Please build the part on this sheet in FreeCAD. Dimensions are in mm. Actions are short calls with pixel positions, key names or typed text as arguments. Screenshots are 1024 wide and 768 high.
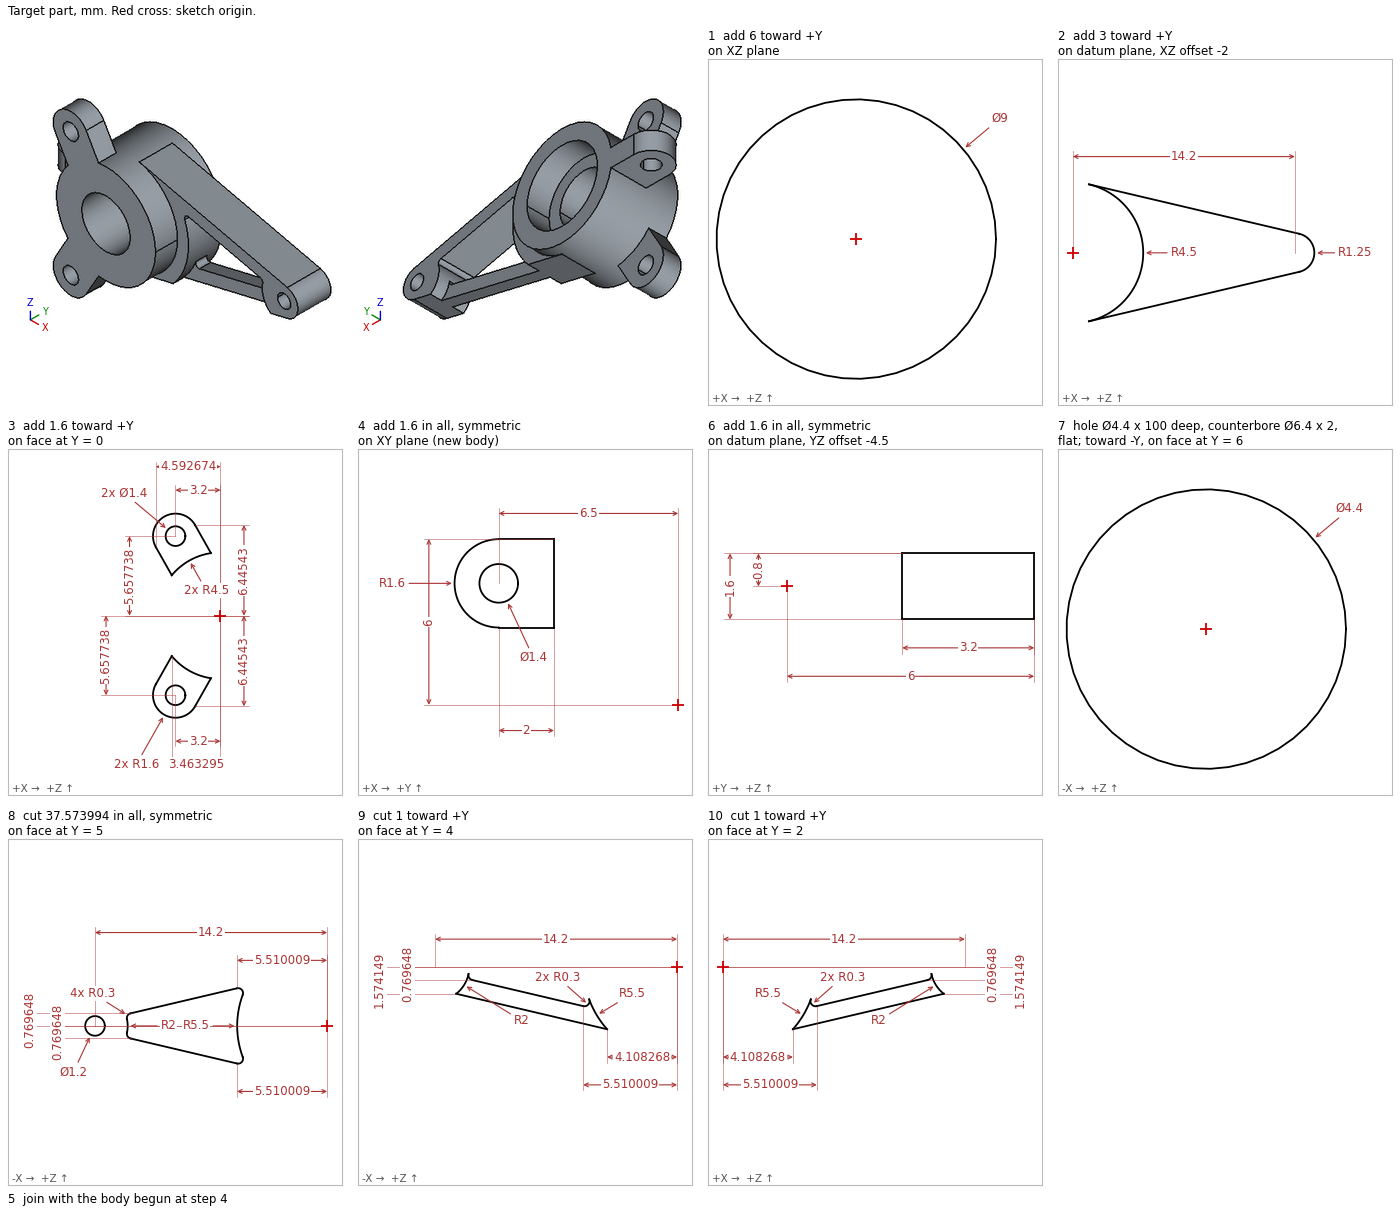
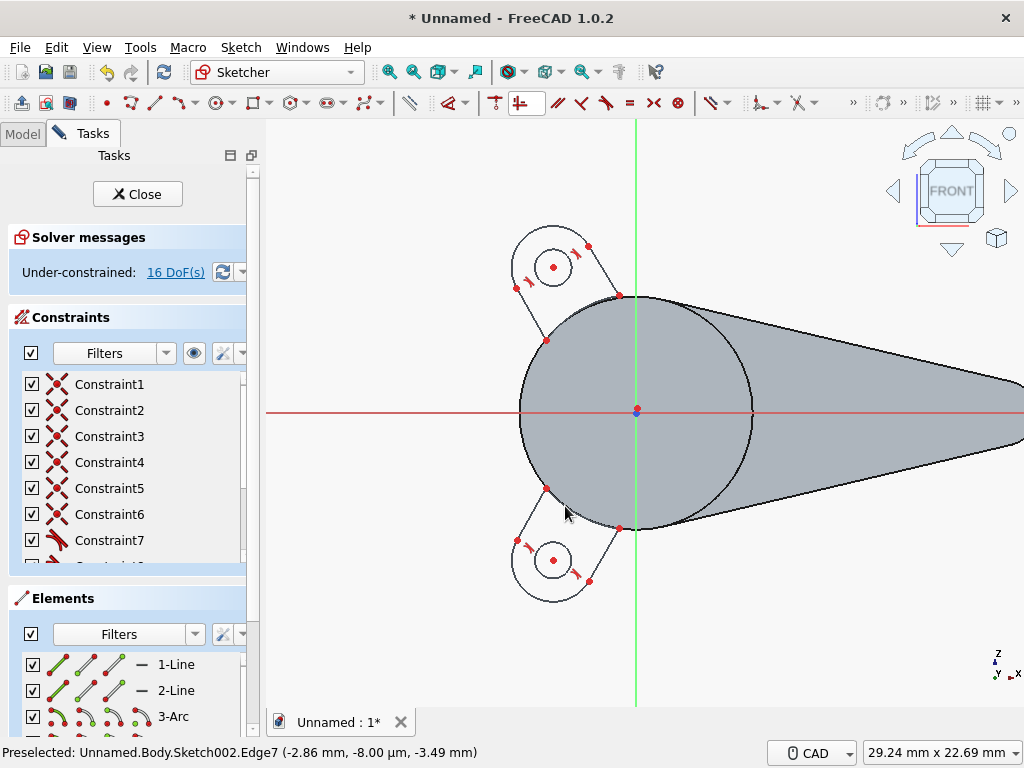
scroll(637, 411, up, 4)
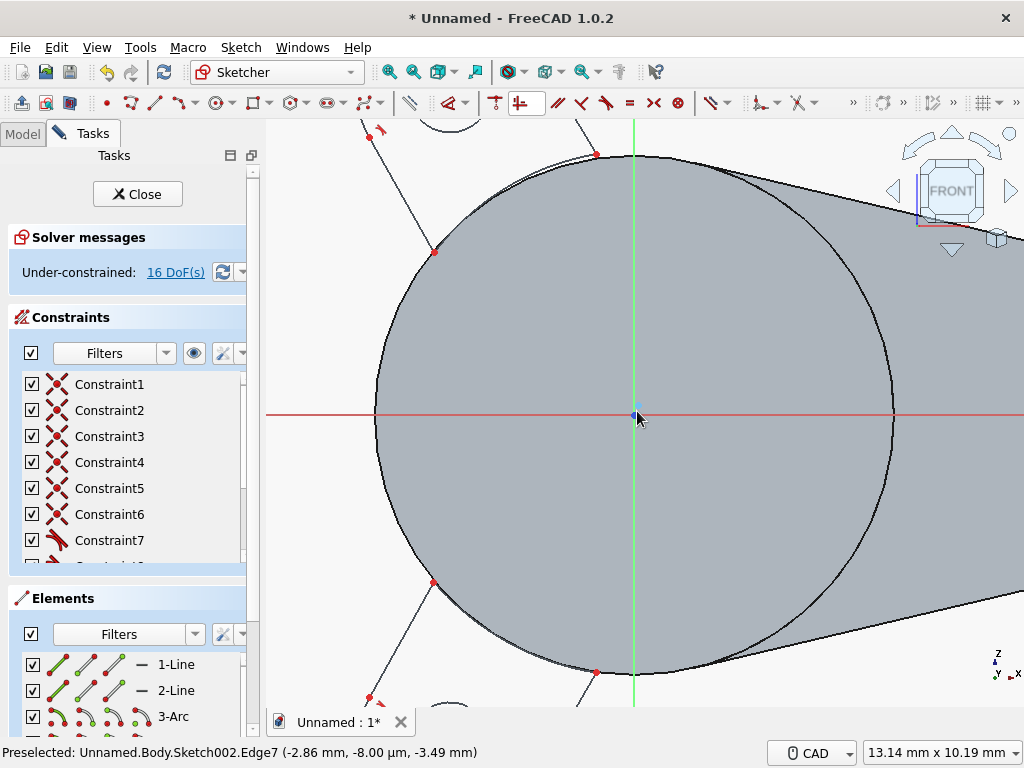
drag(624, 396, 648, 425)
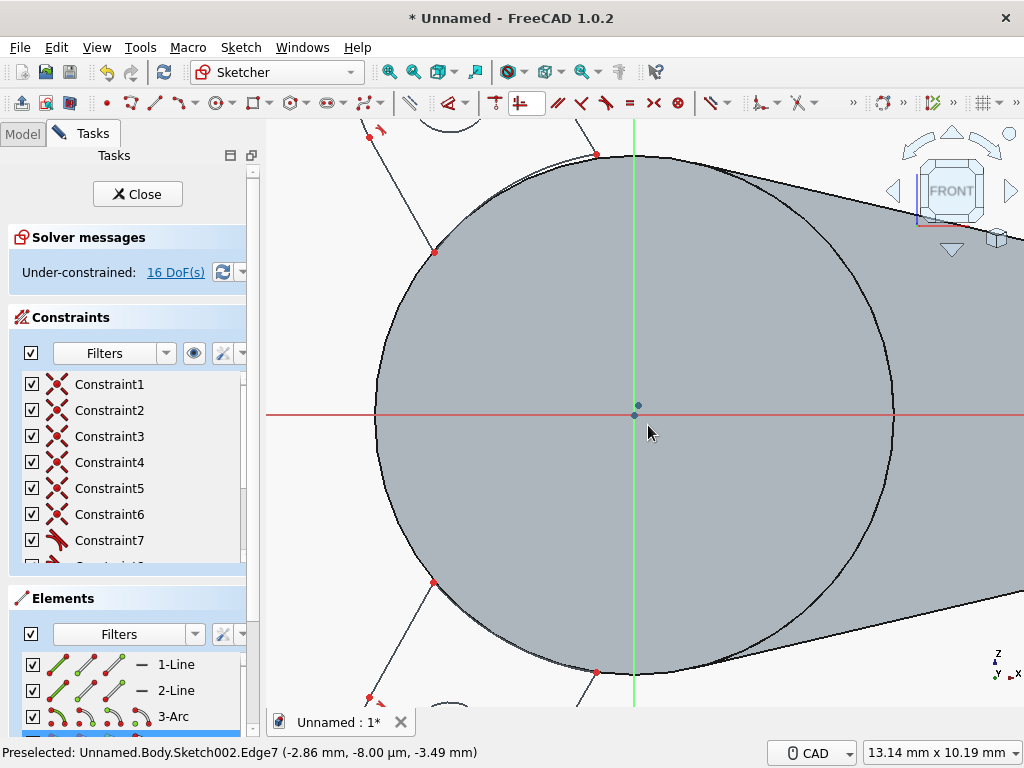
key(c)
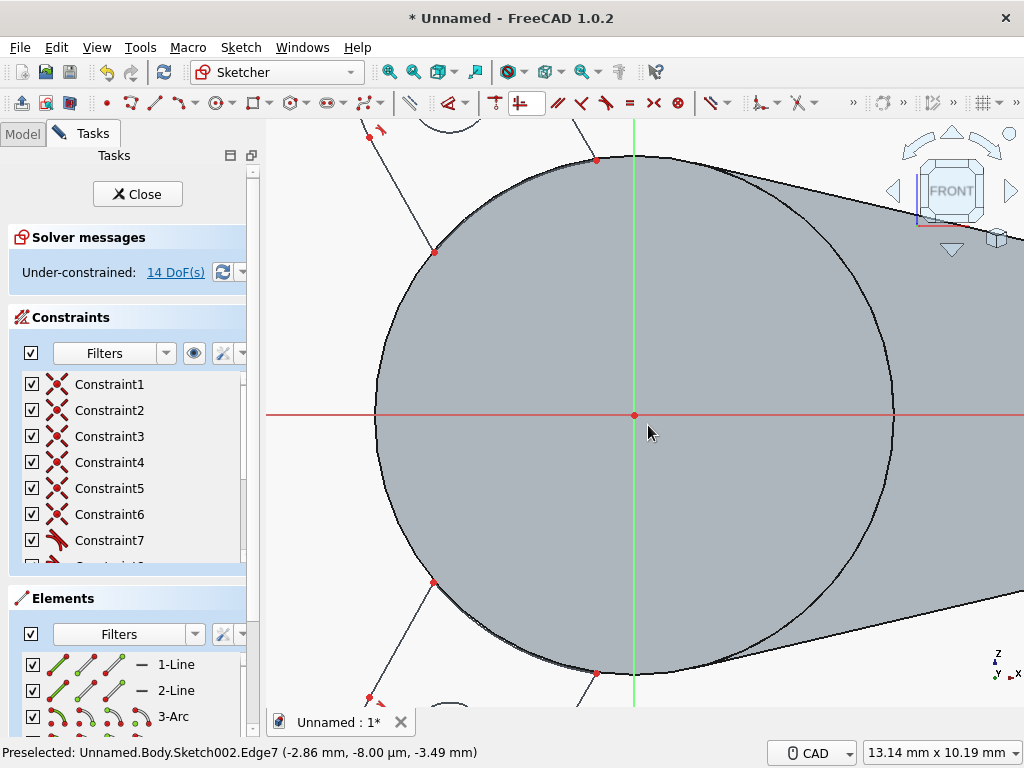
click(541, 175)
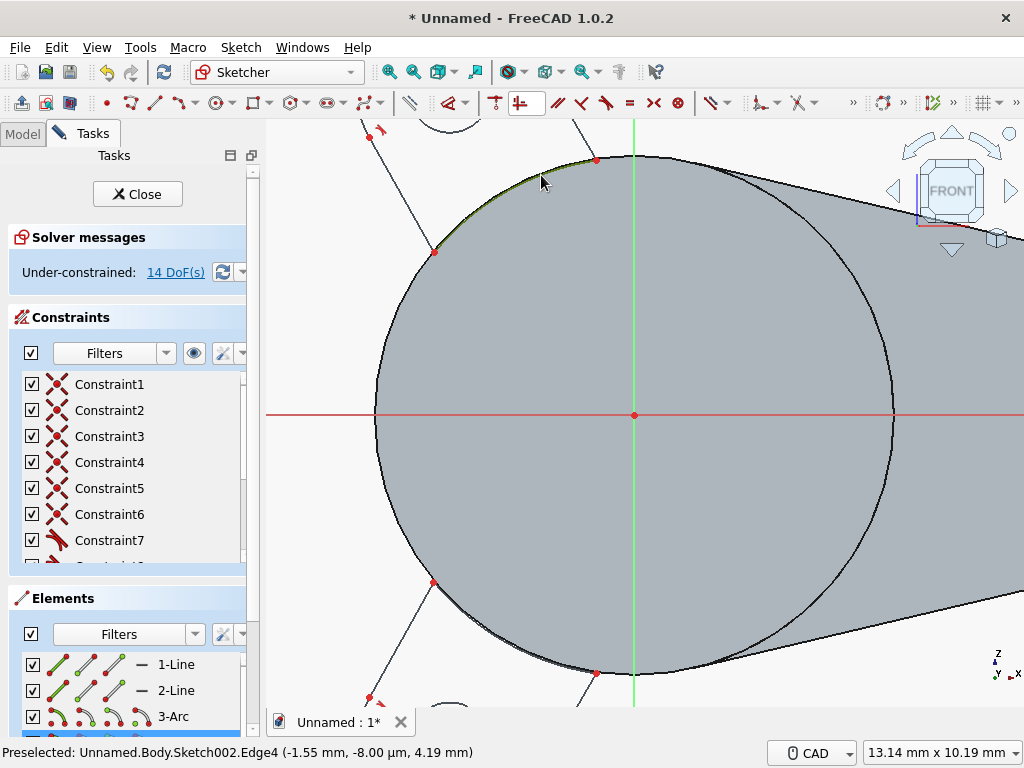
click(475, 622)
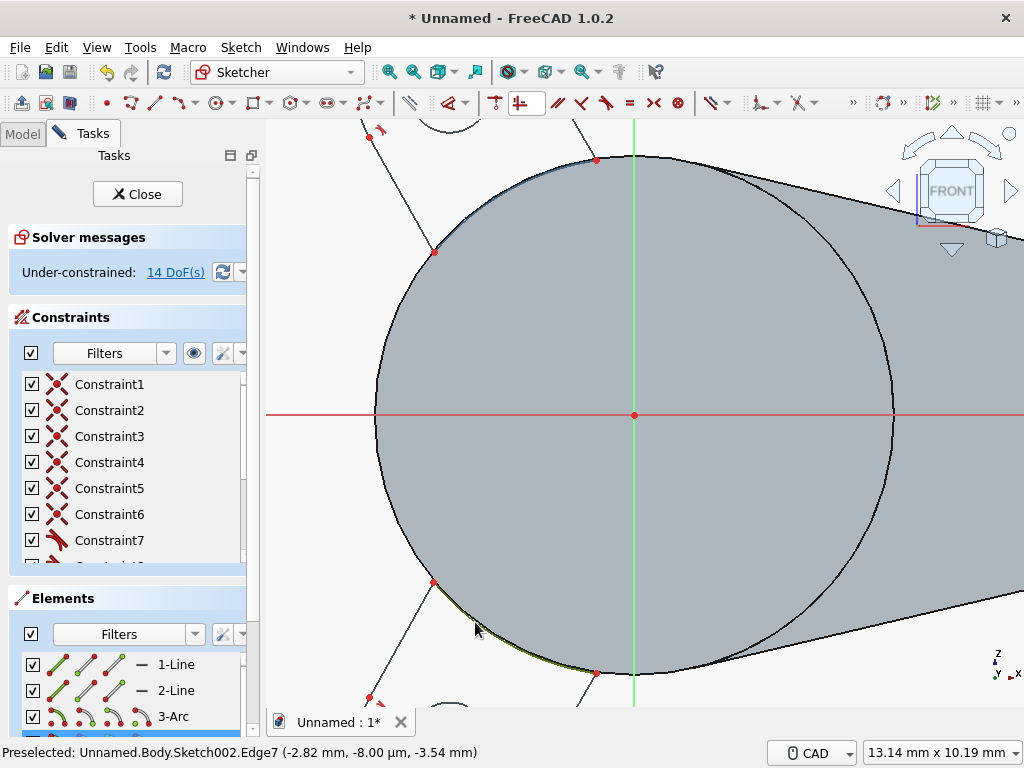
key(e)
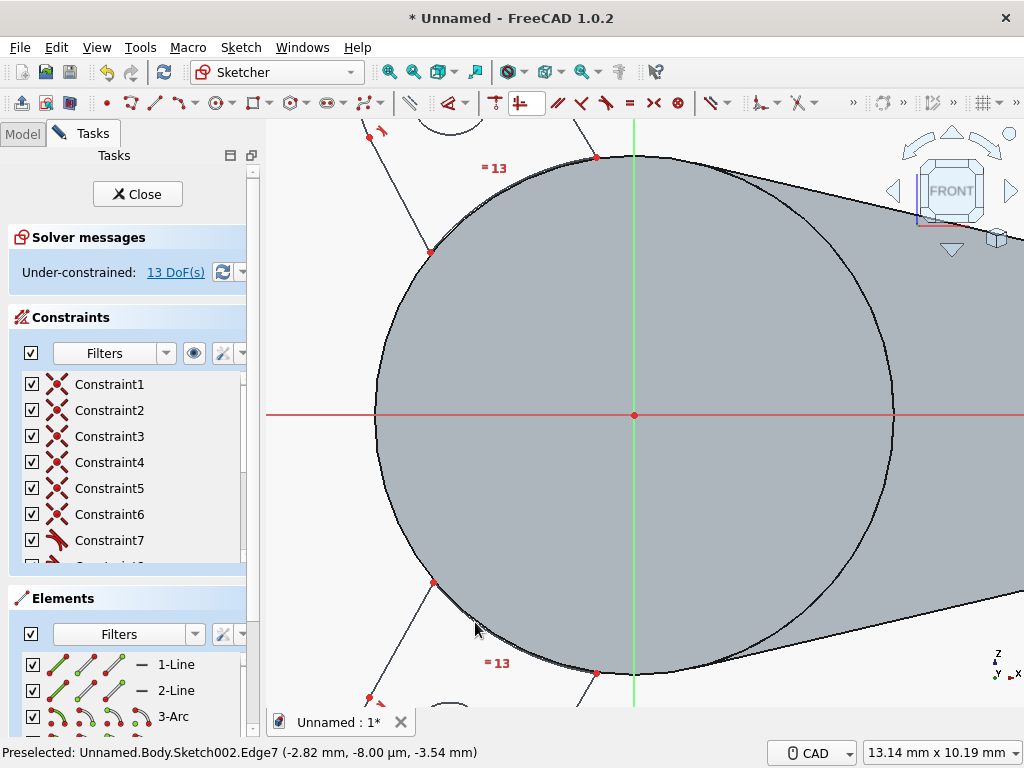
scroll(637, 411, down, 4)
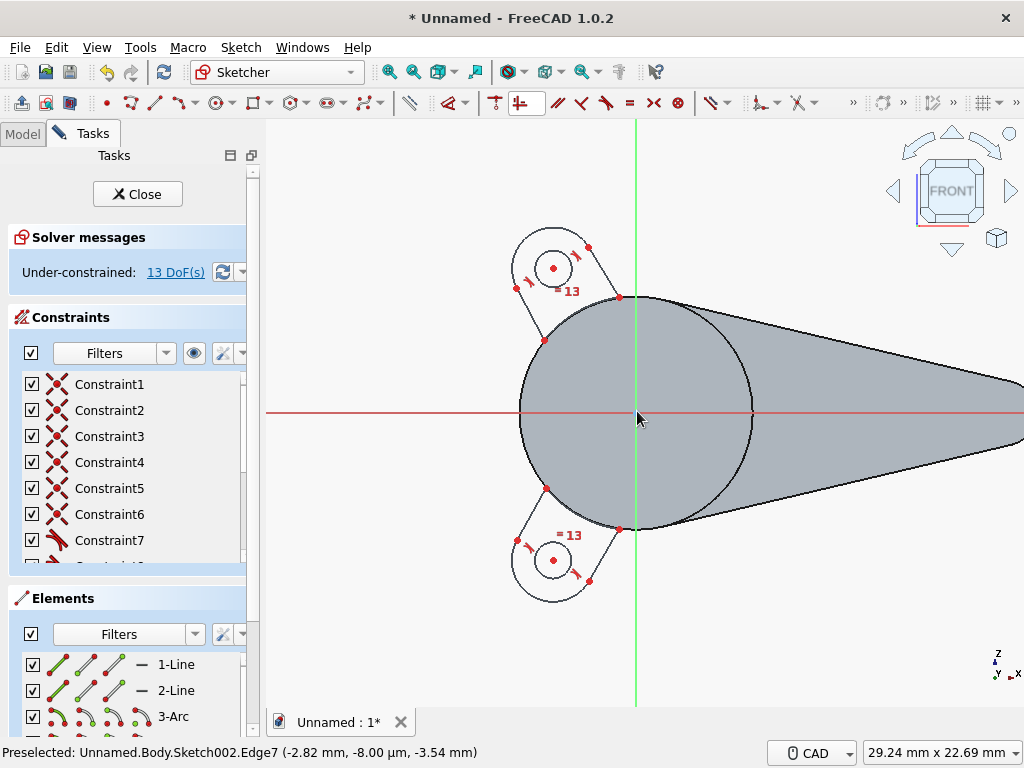
click(558, 228)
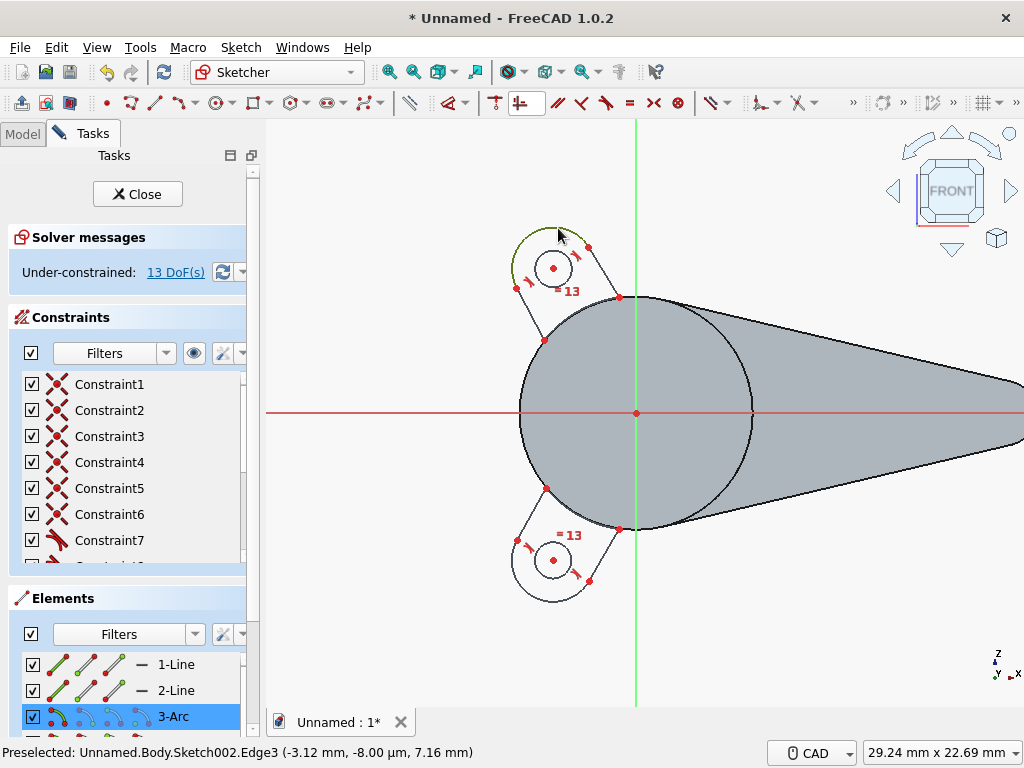
click(516, 578)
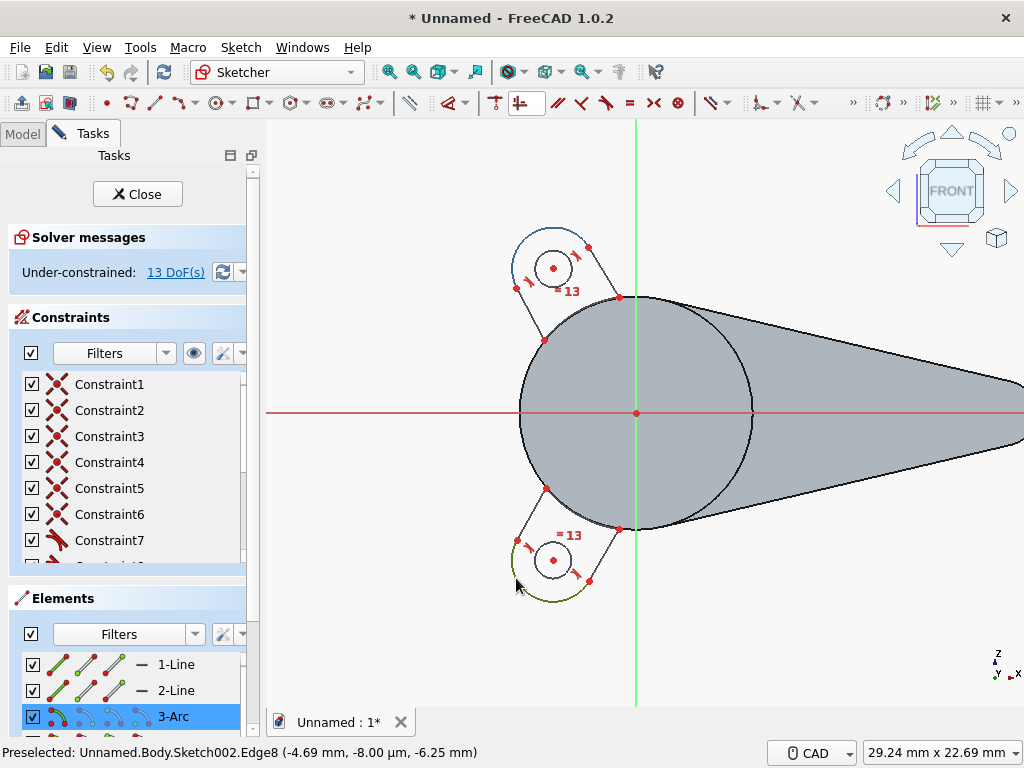
click(630, 104)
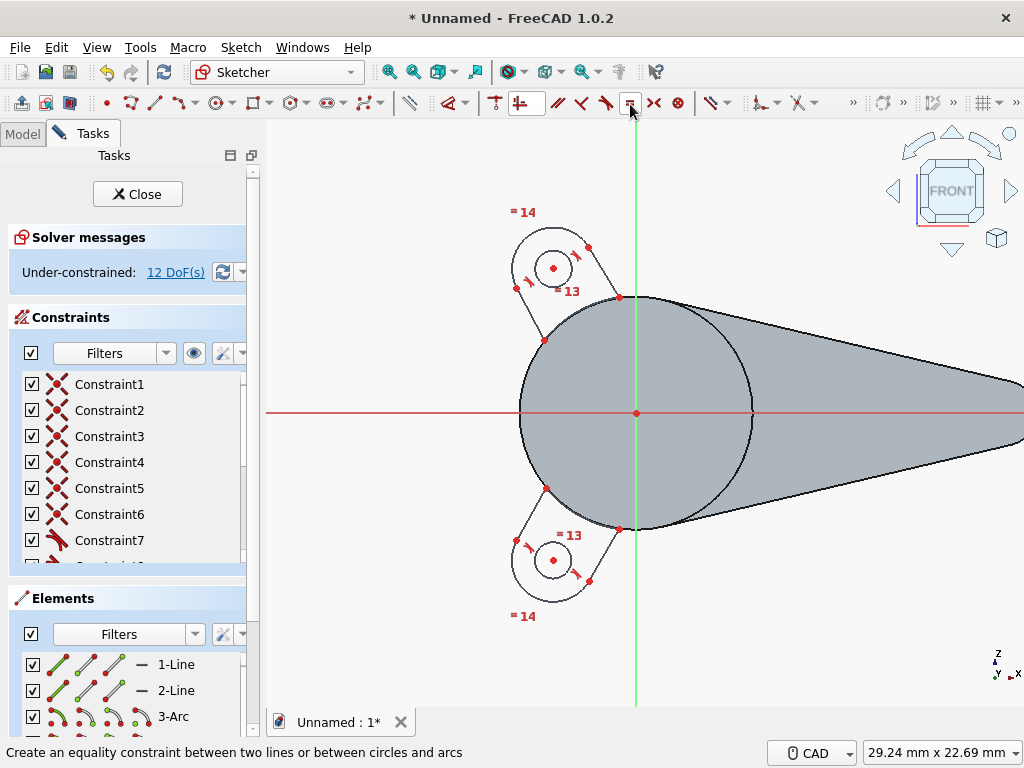
click(566, 256)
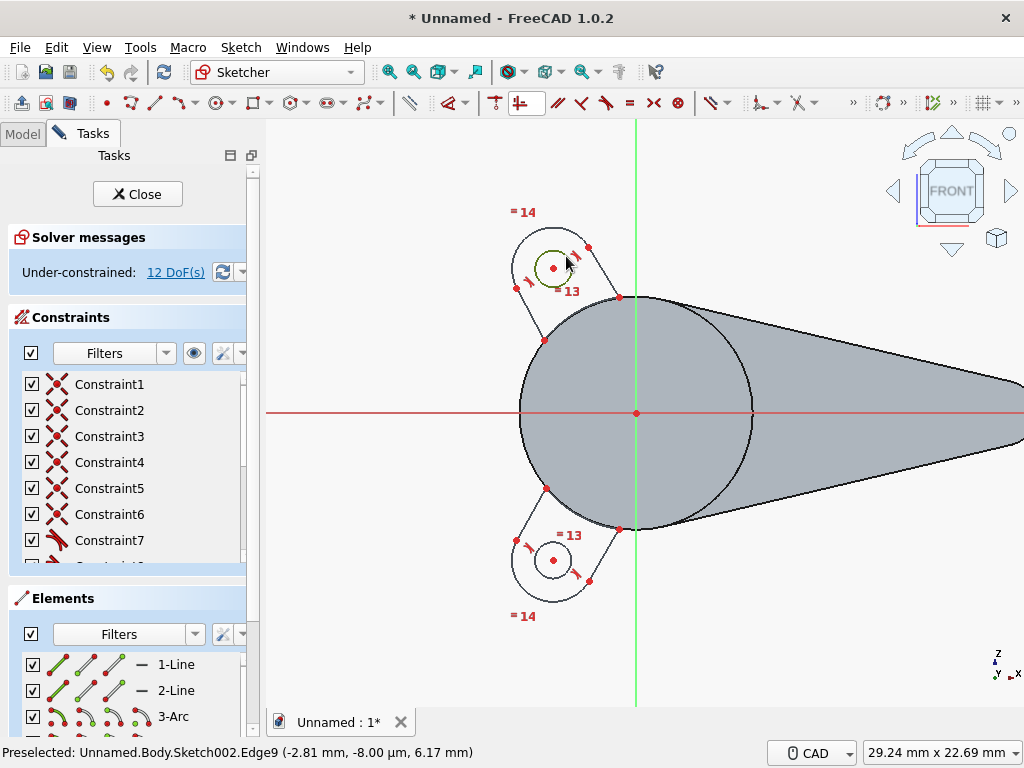
click(566, 548)